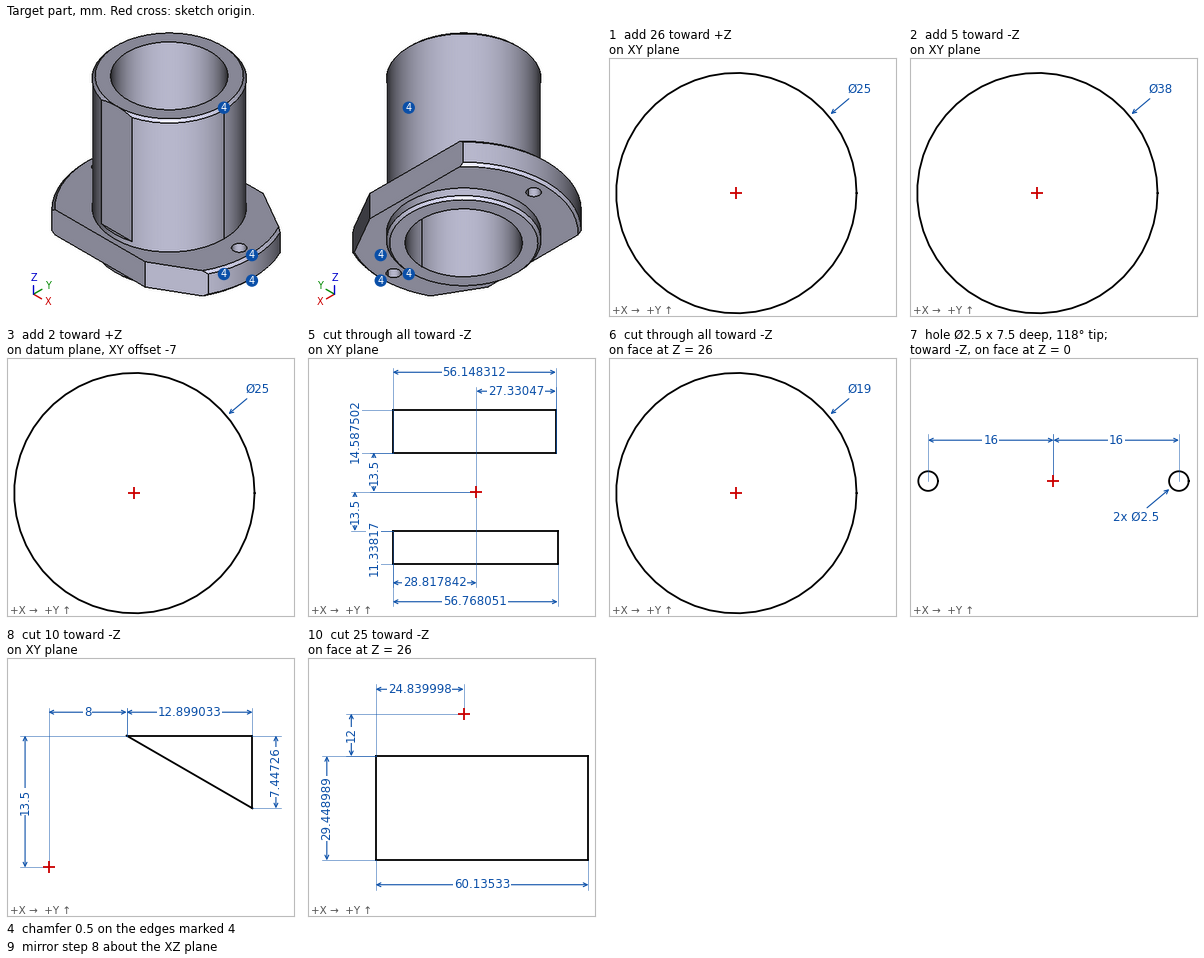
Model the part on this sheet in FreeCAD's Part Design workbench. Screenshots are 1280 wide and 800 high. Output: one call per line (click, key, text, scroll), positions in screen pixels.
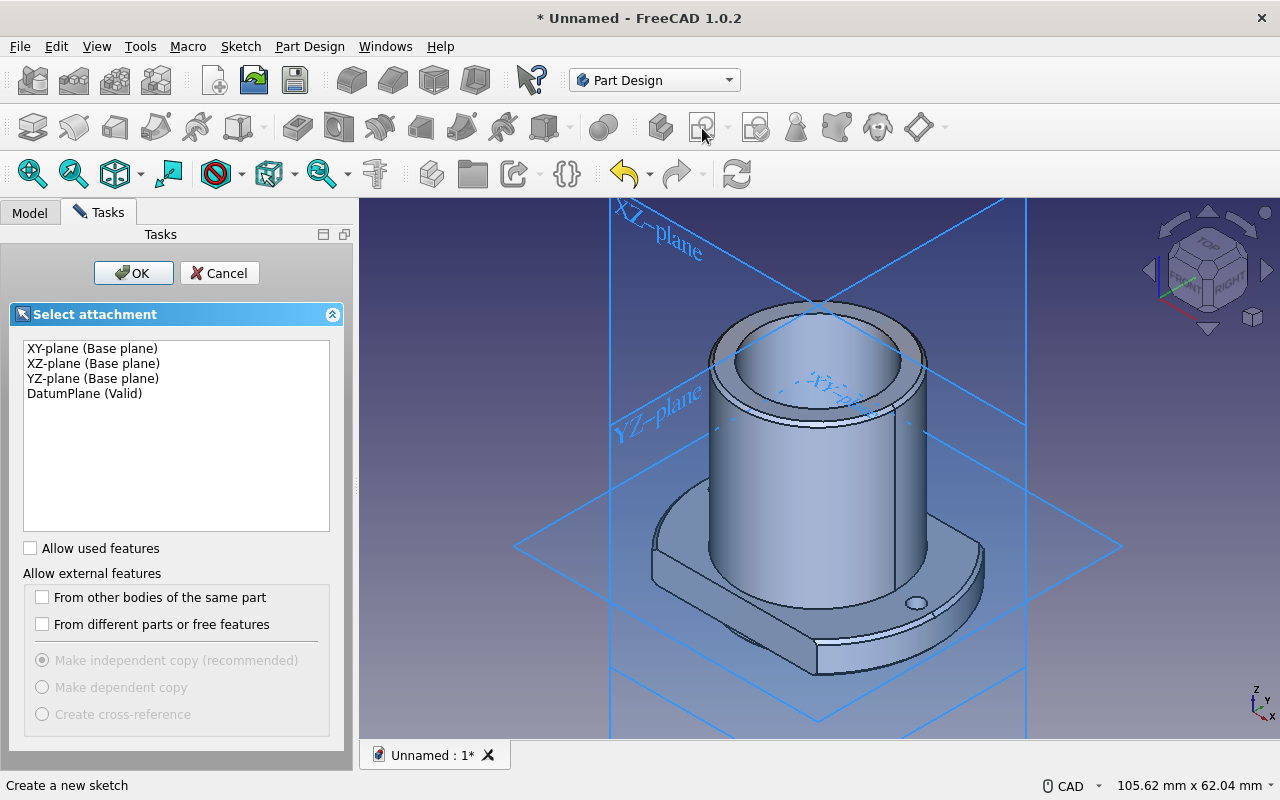
click(84, 348)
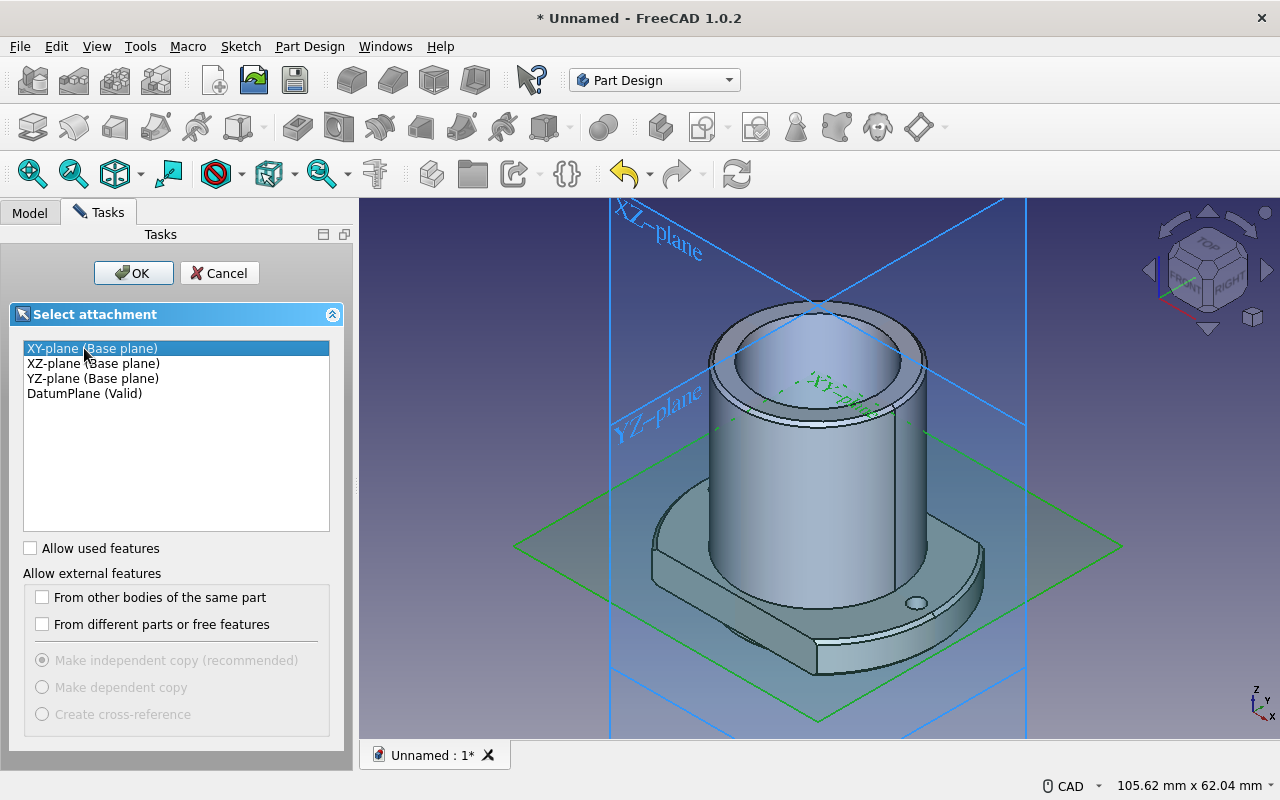
click(134, 273)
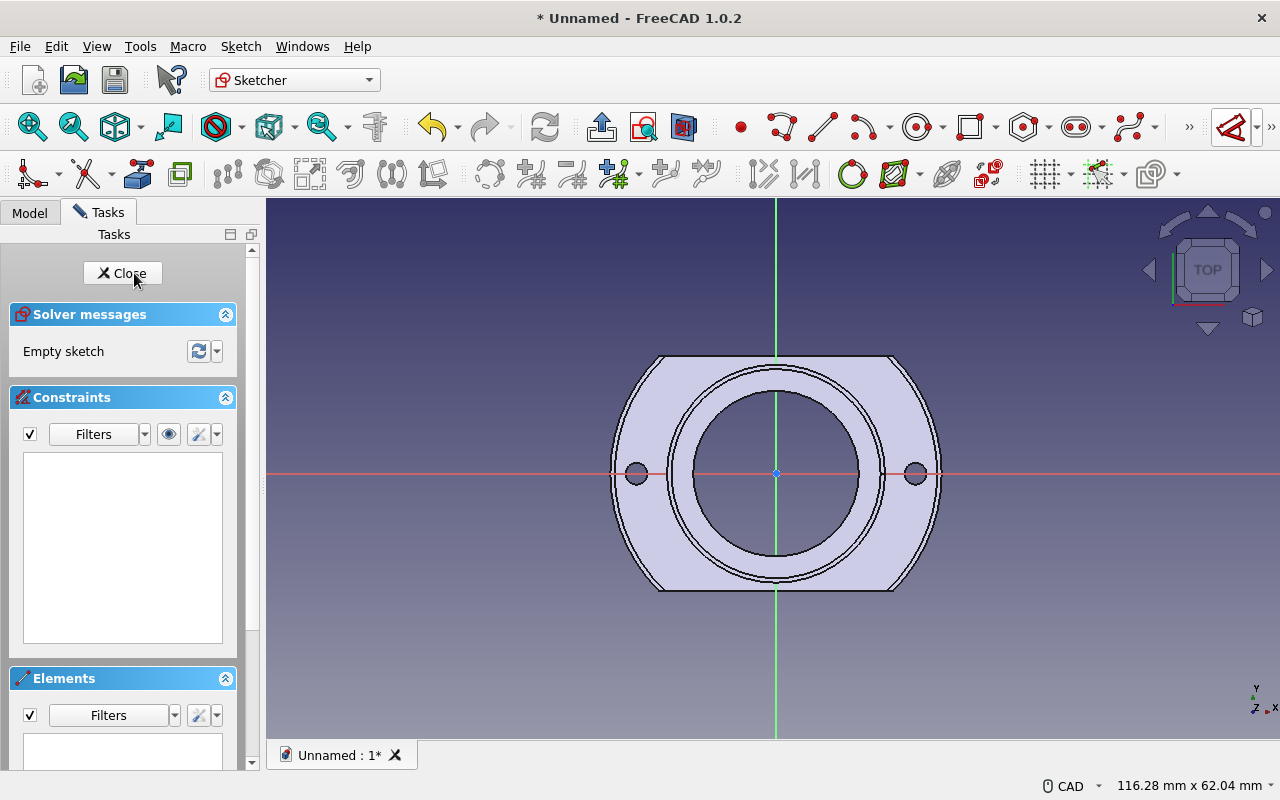
click(684, 128)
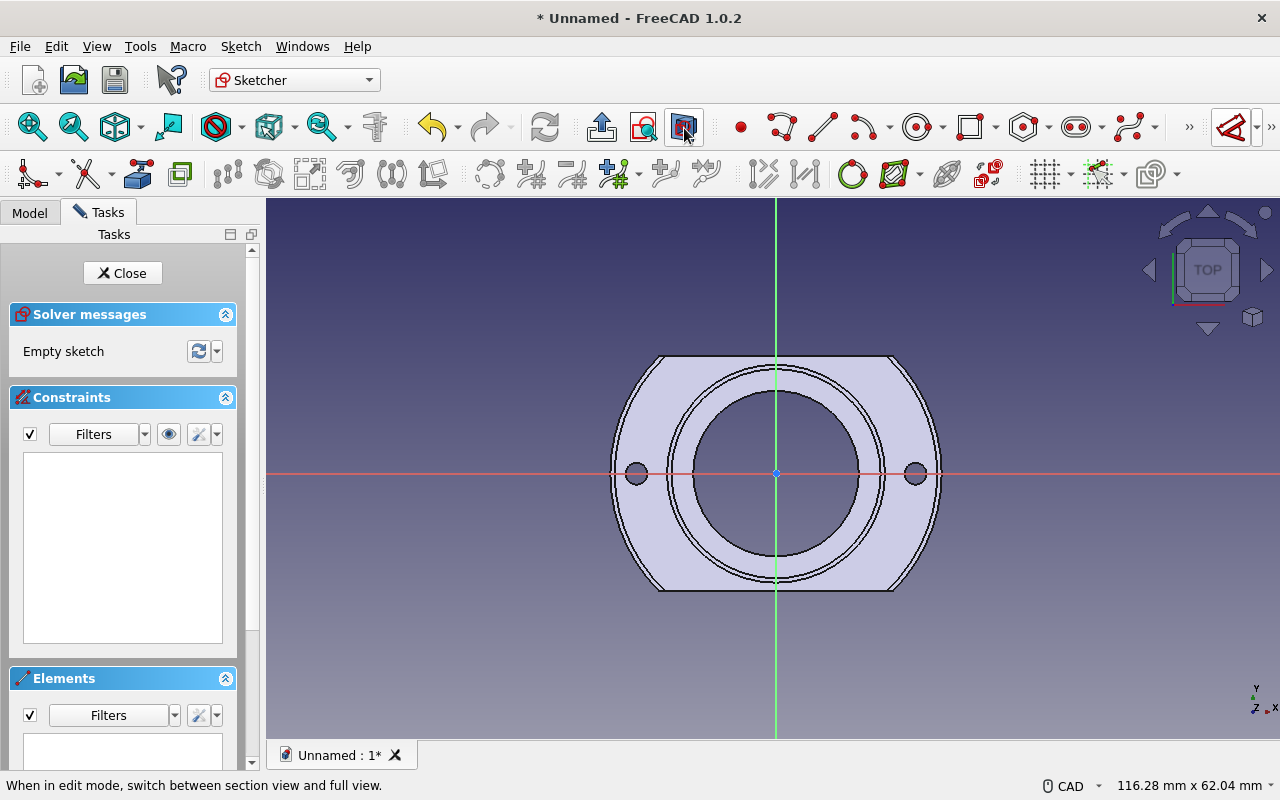
scroll(962, 384, up, 5)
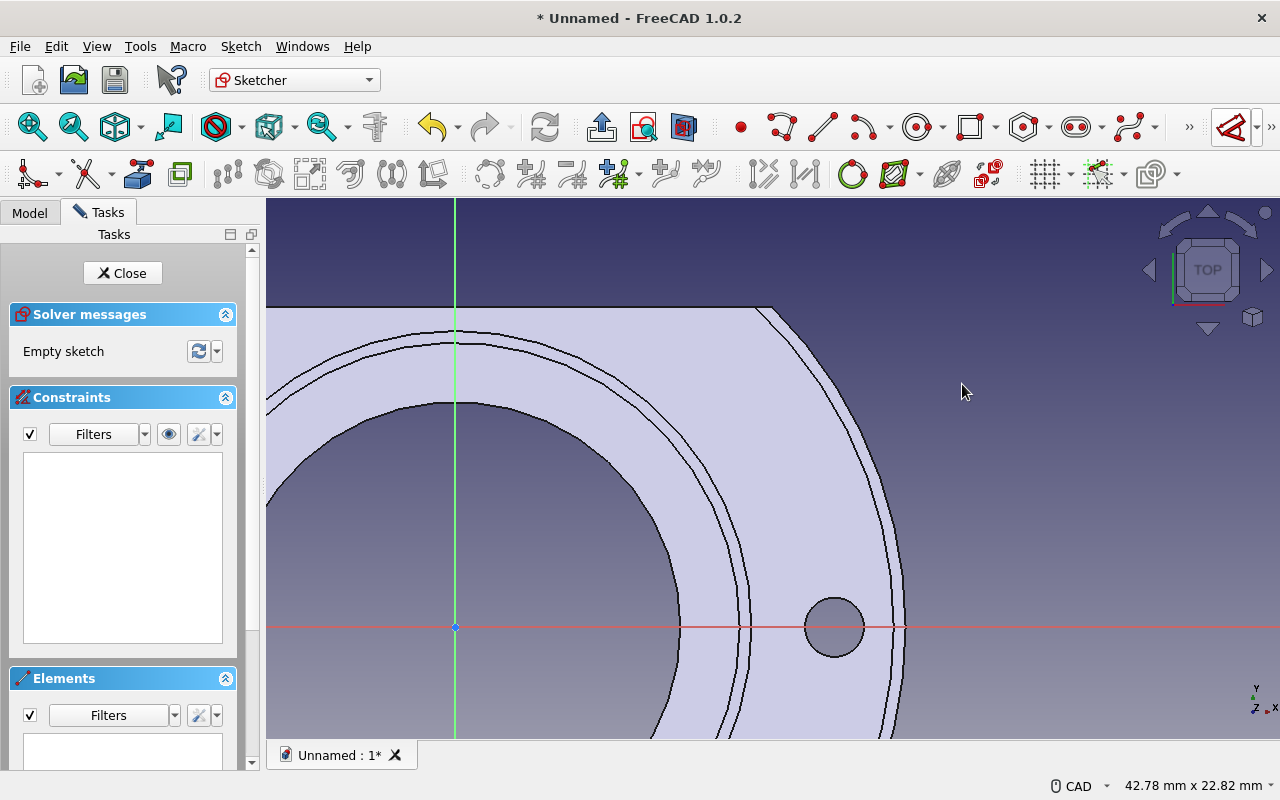
click(782, 128)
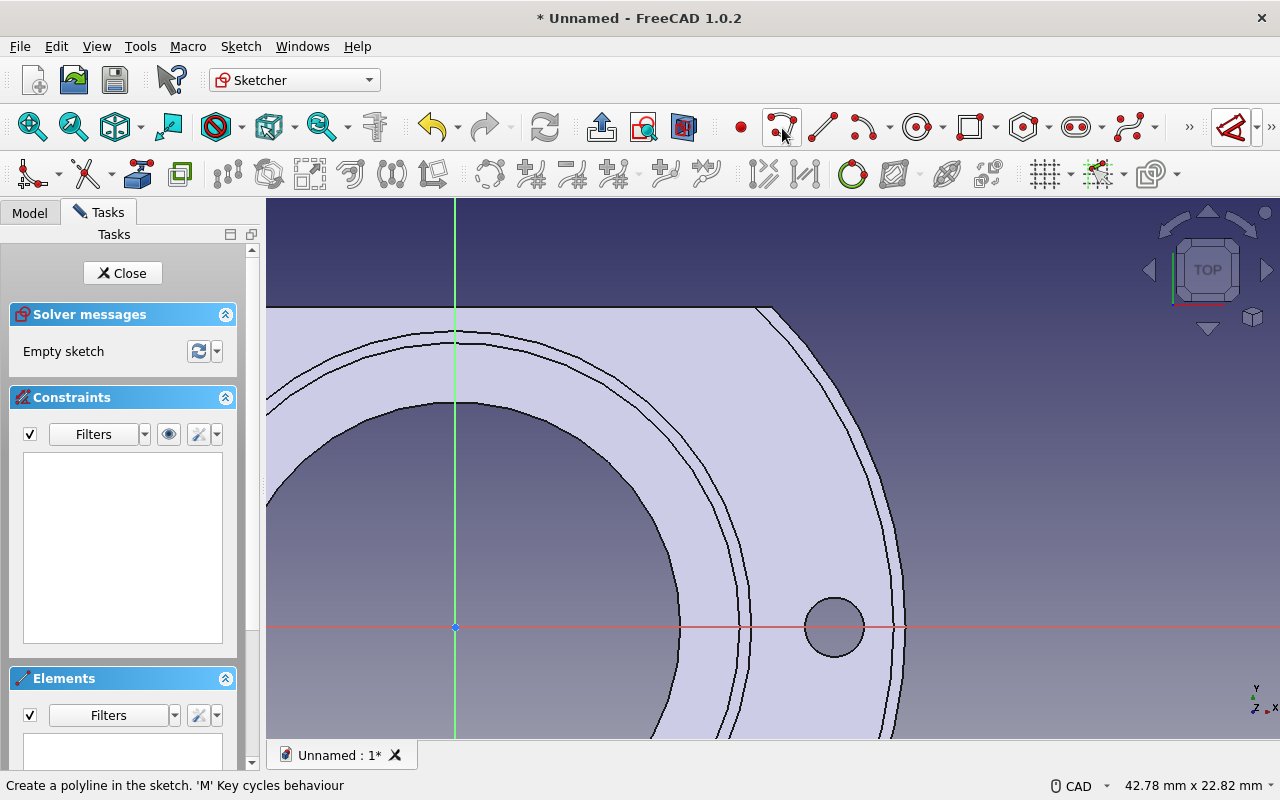
click(645, 307)
click(951, 484)
click(951, 307)
click(645, 308)
key(Escape)
key(Escape)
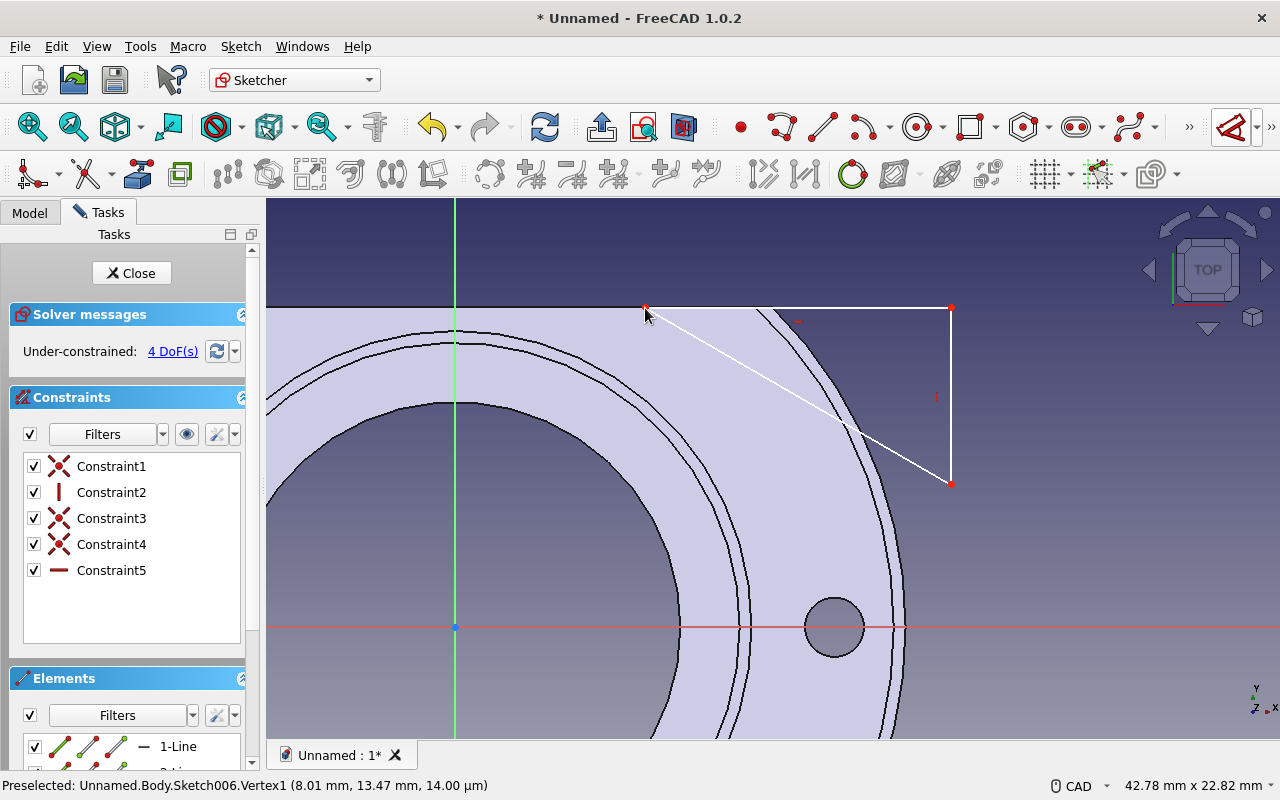
click(645, 308)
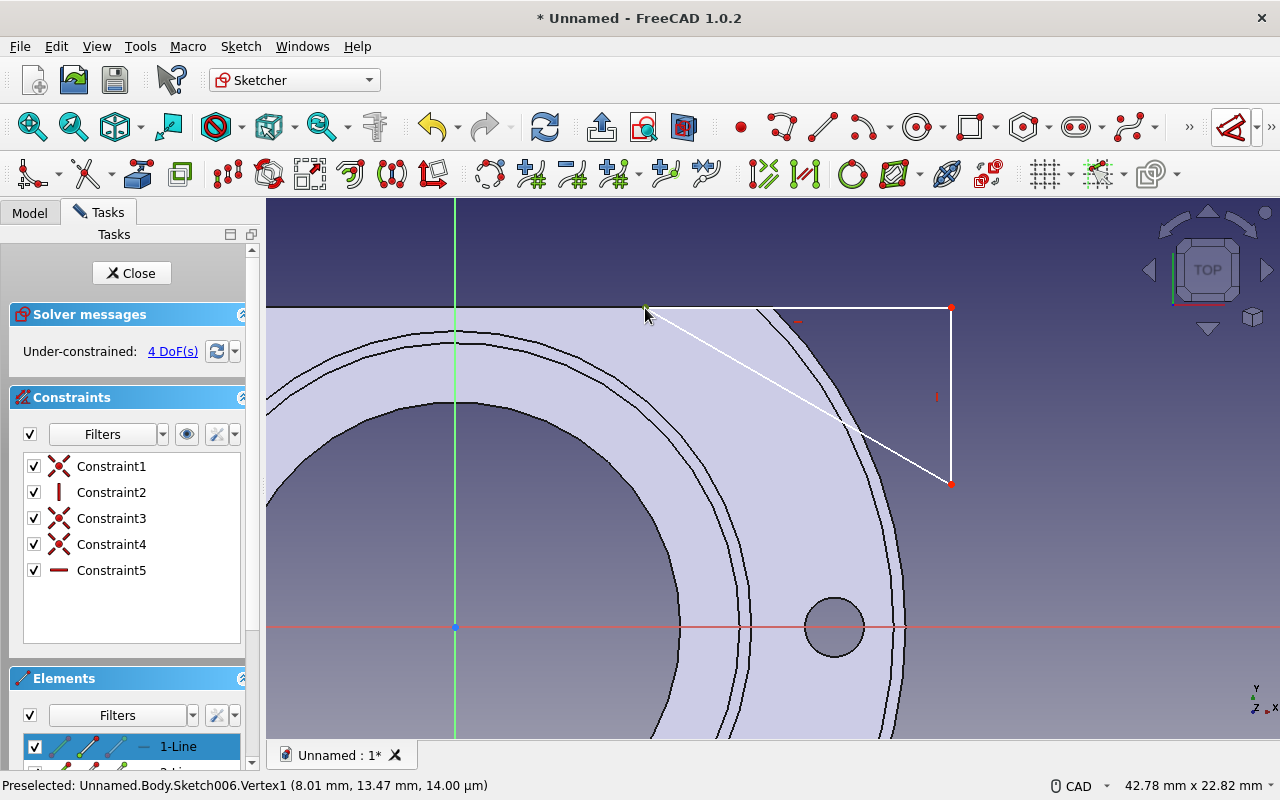
click(1256, 128)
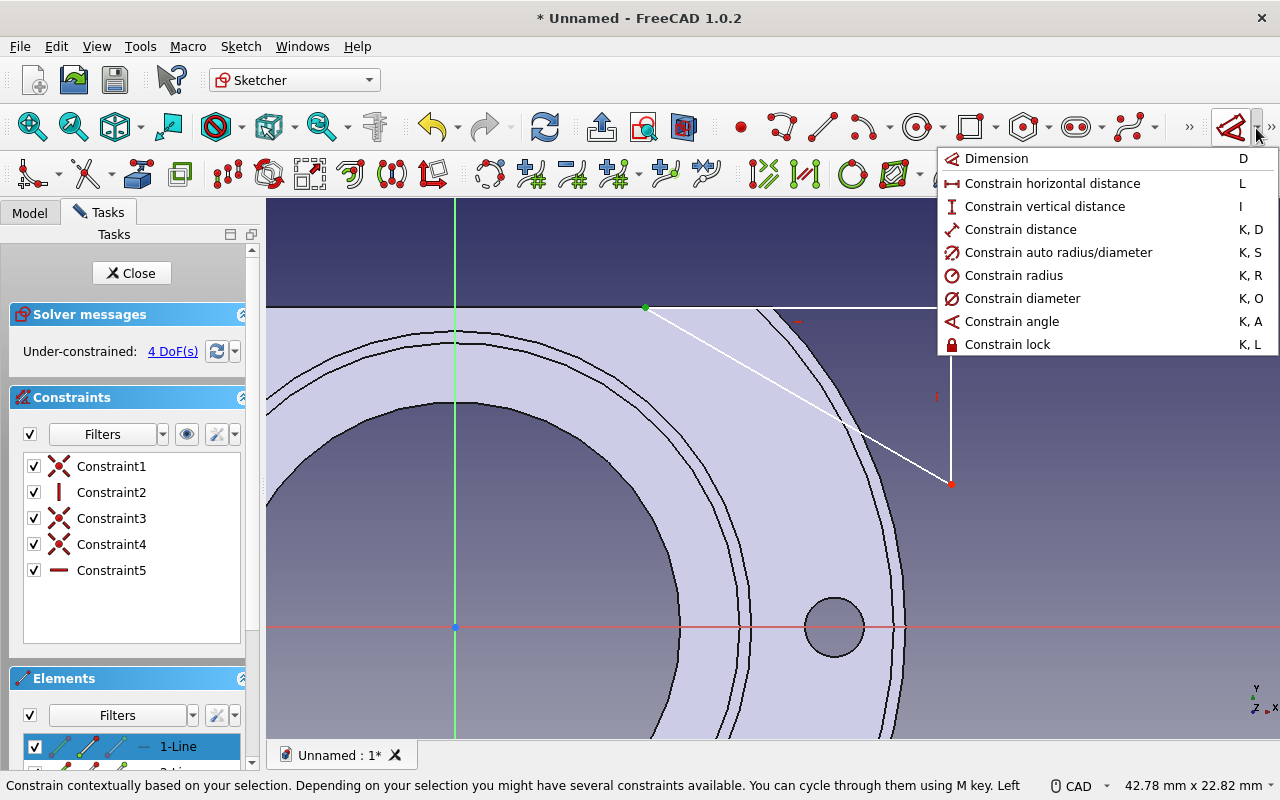
click(1108, 184)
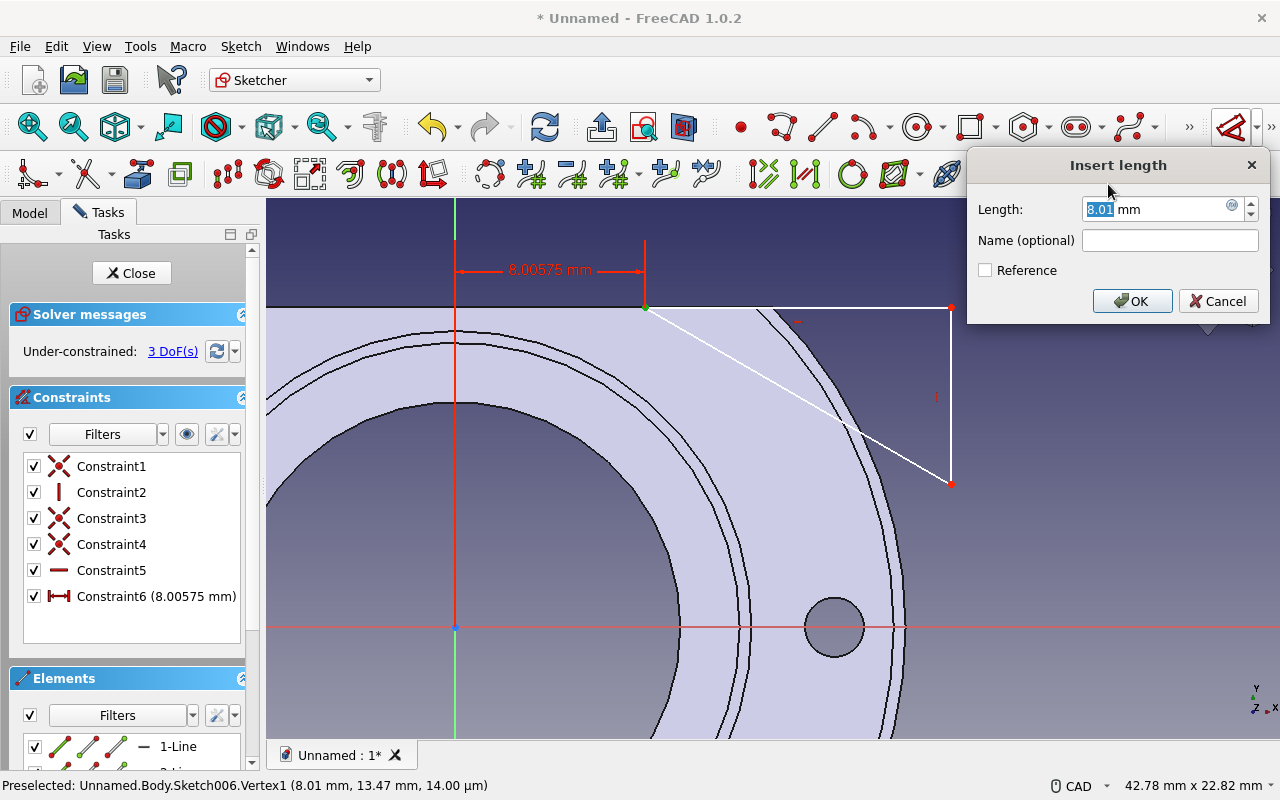
text(8)
key(Return)